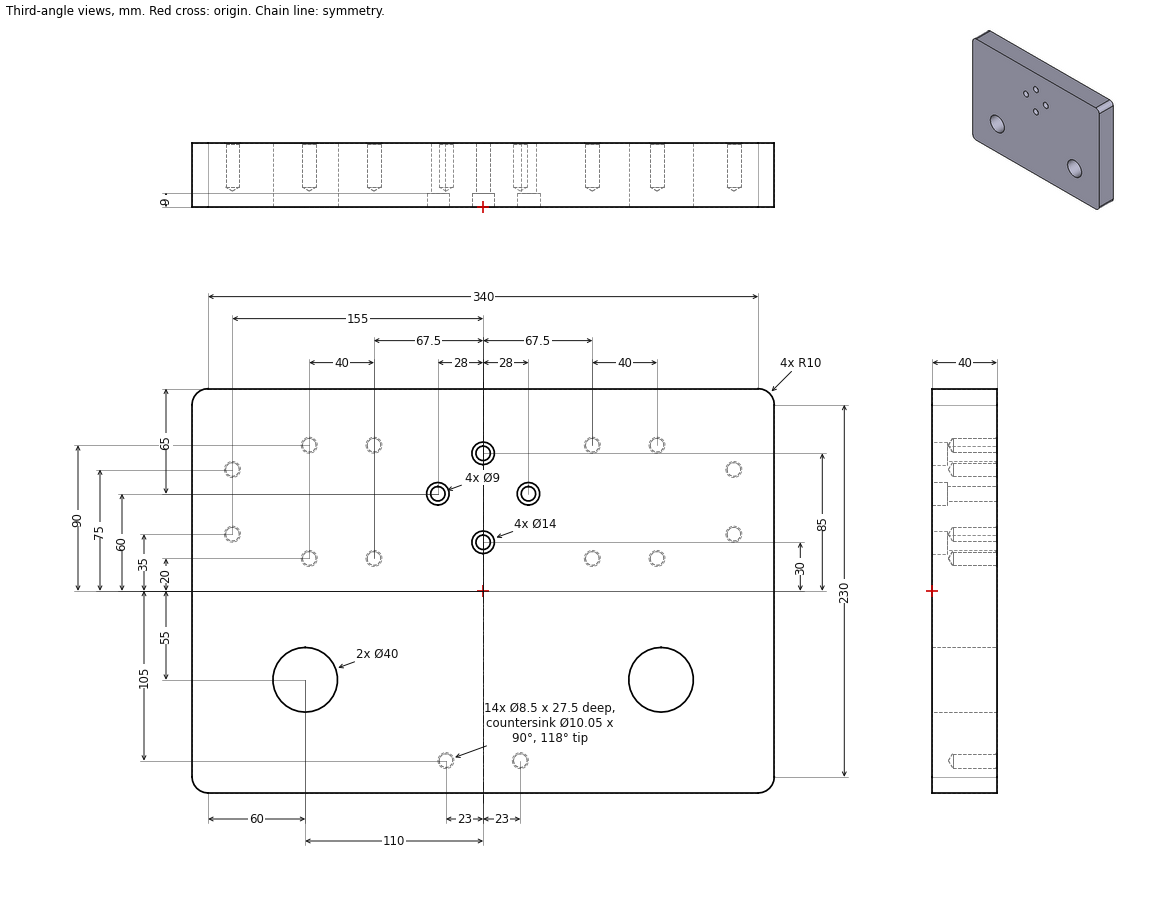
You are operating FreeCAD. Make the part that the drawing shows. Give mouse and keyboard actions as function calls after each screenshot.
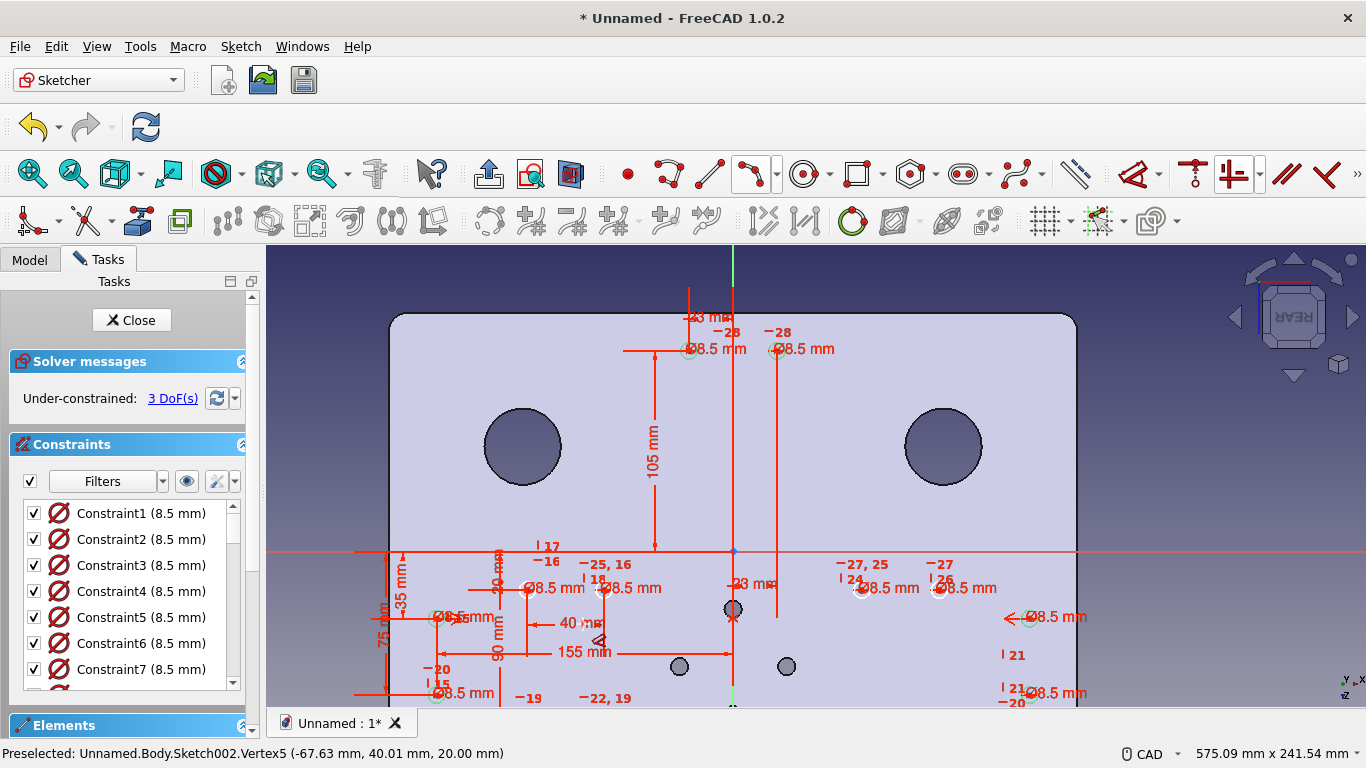
scroll(777, 351, down, 2)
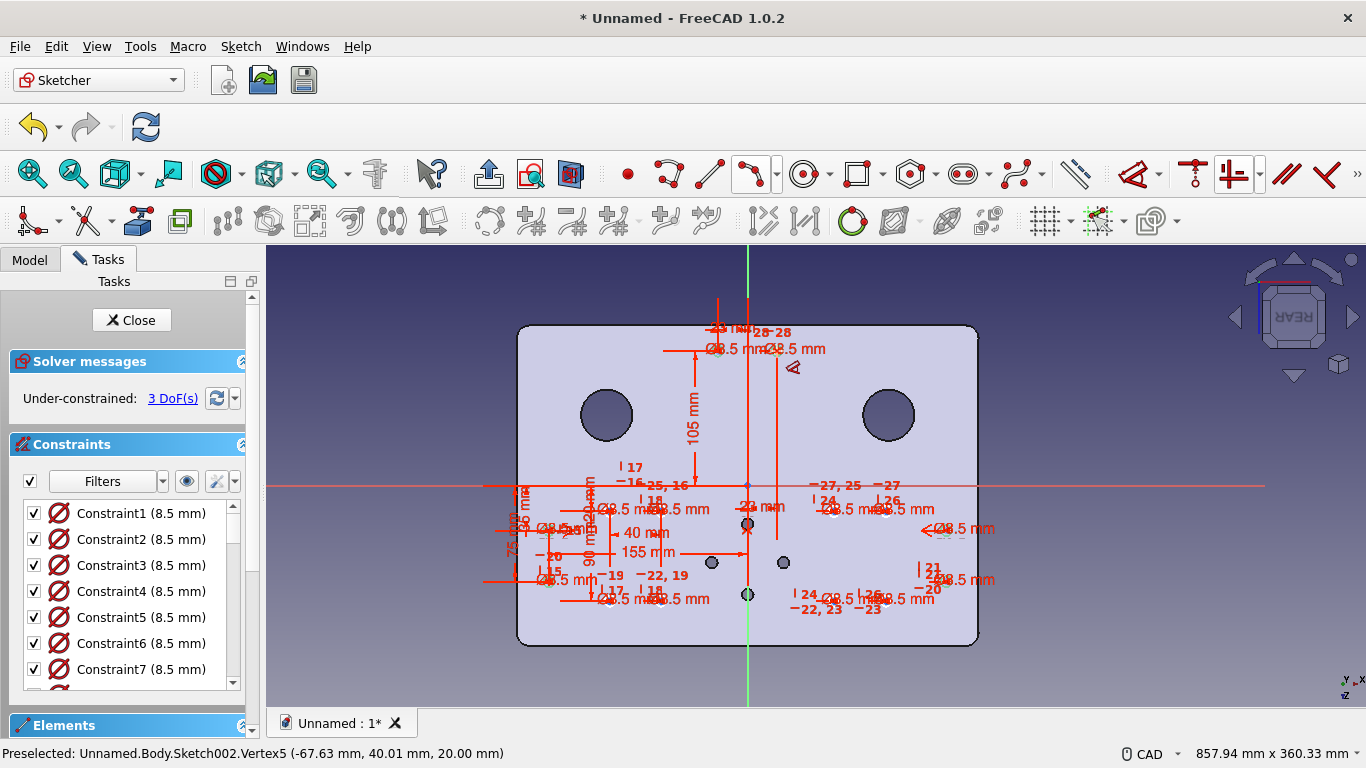
click(834, 601)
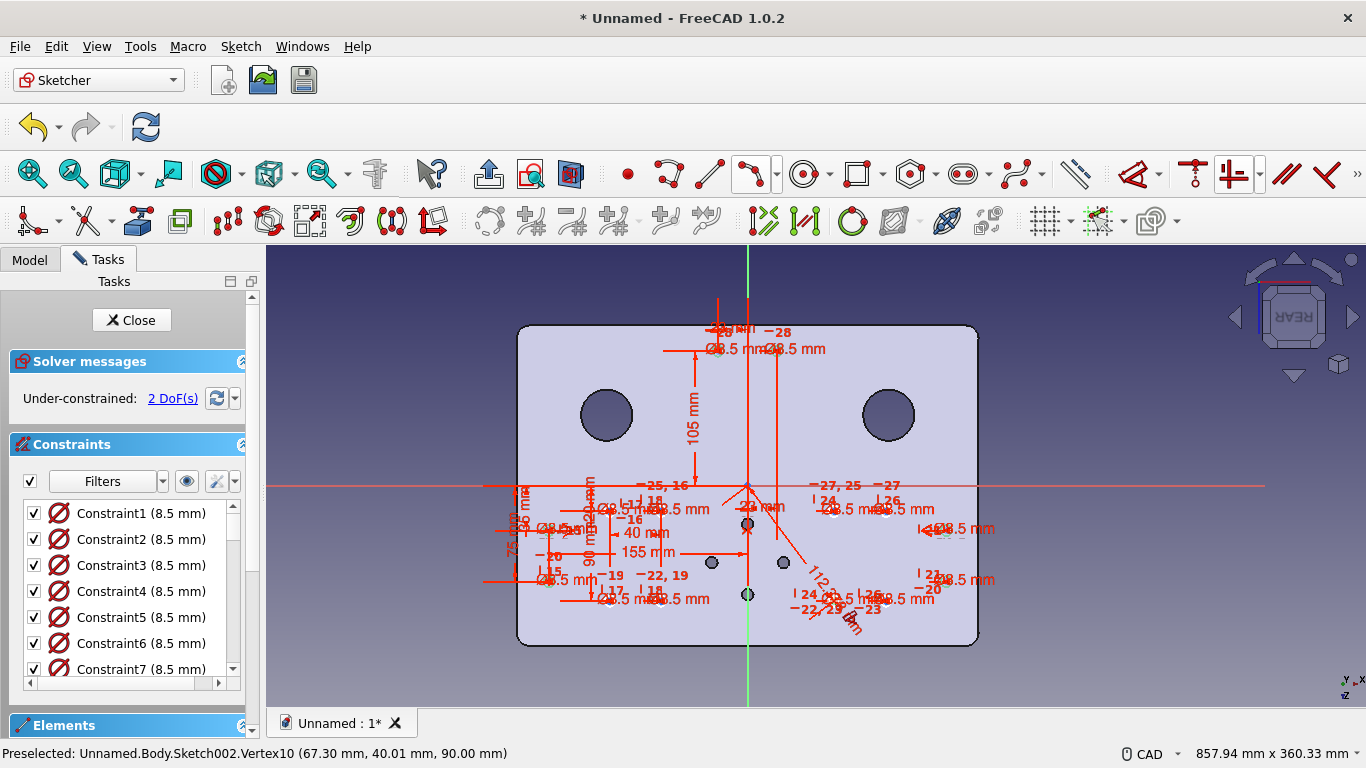
click(886, 601)
click(860, 635)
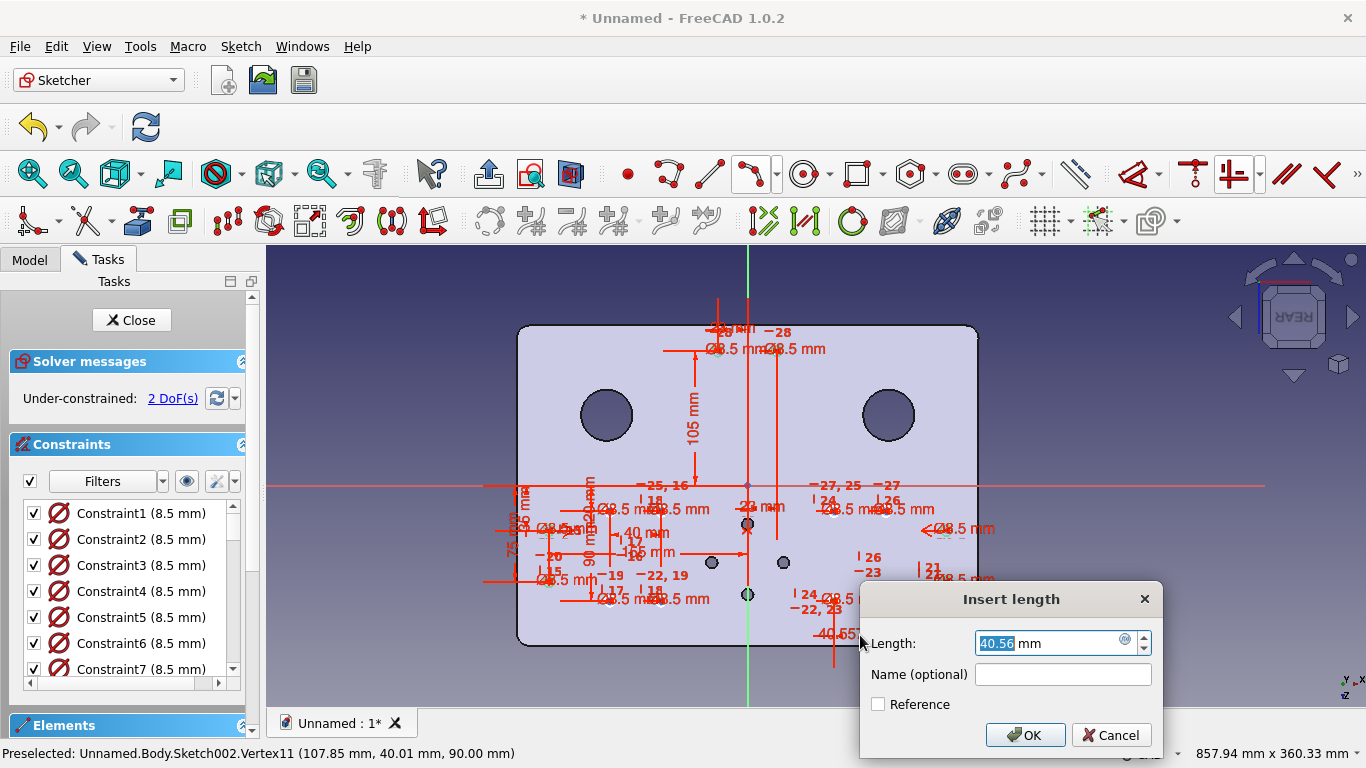
text(40)
key(Return)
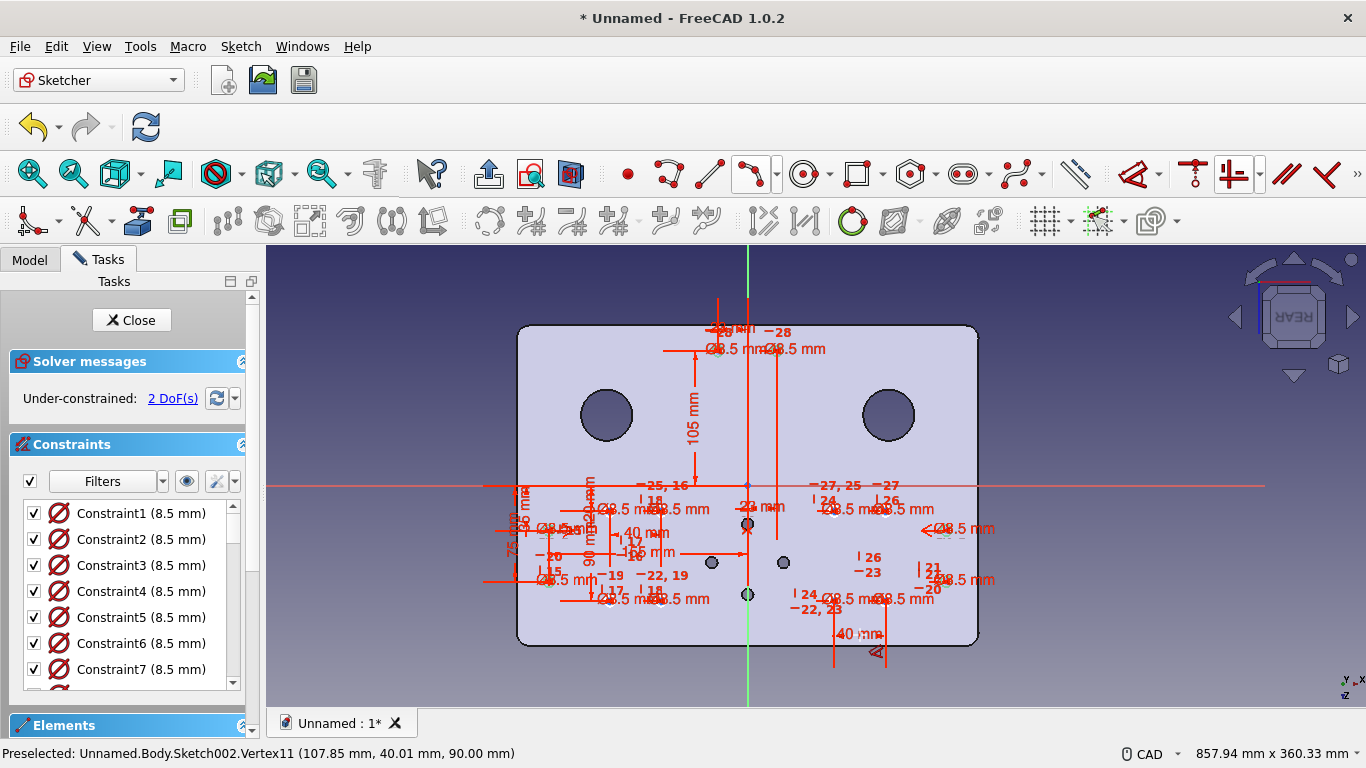
click(661, 511)
click(724, 545)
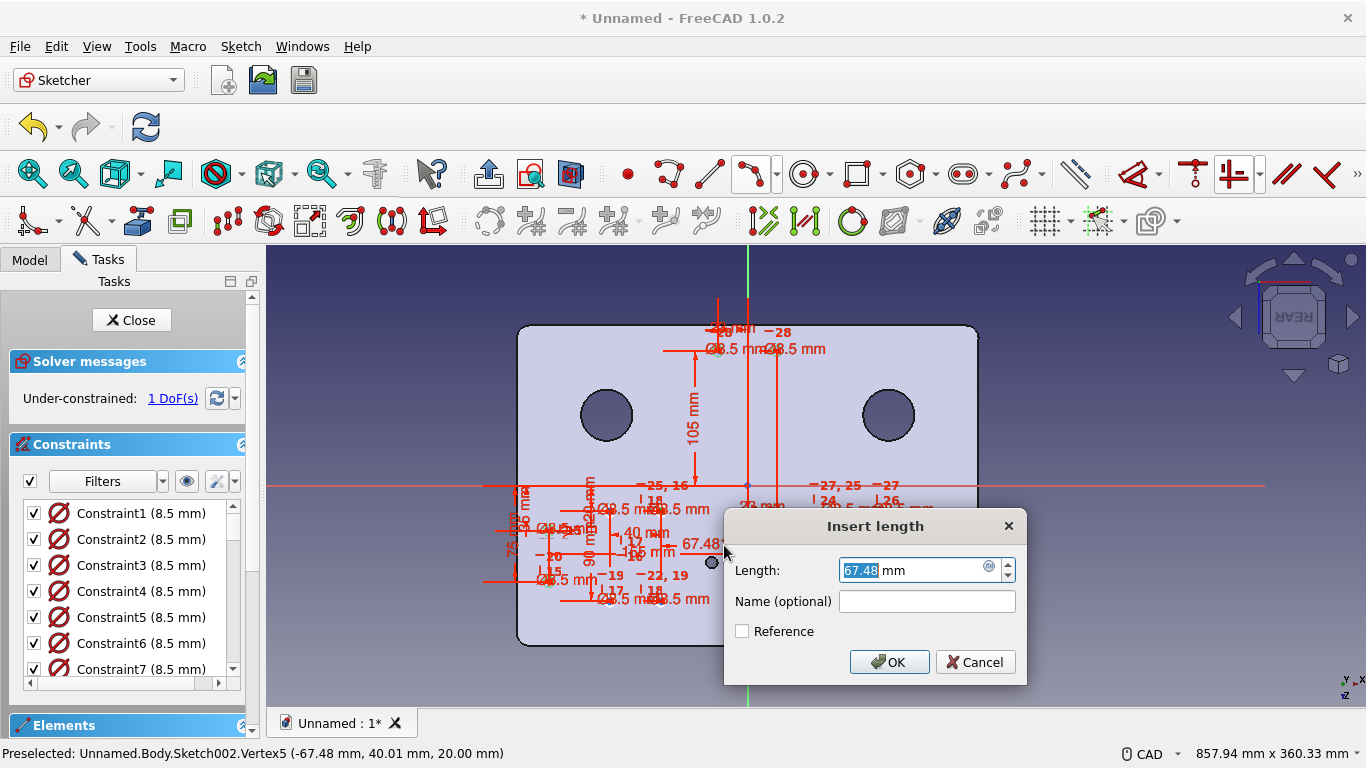
text(67.5)
key(Return)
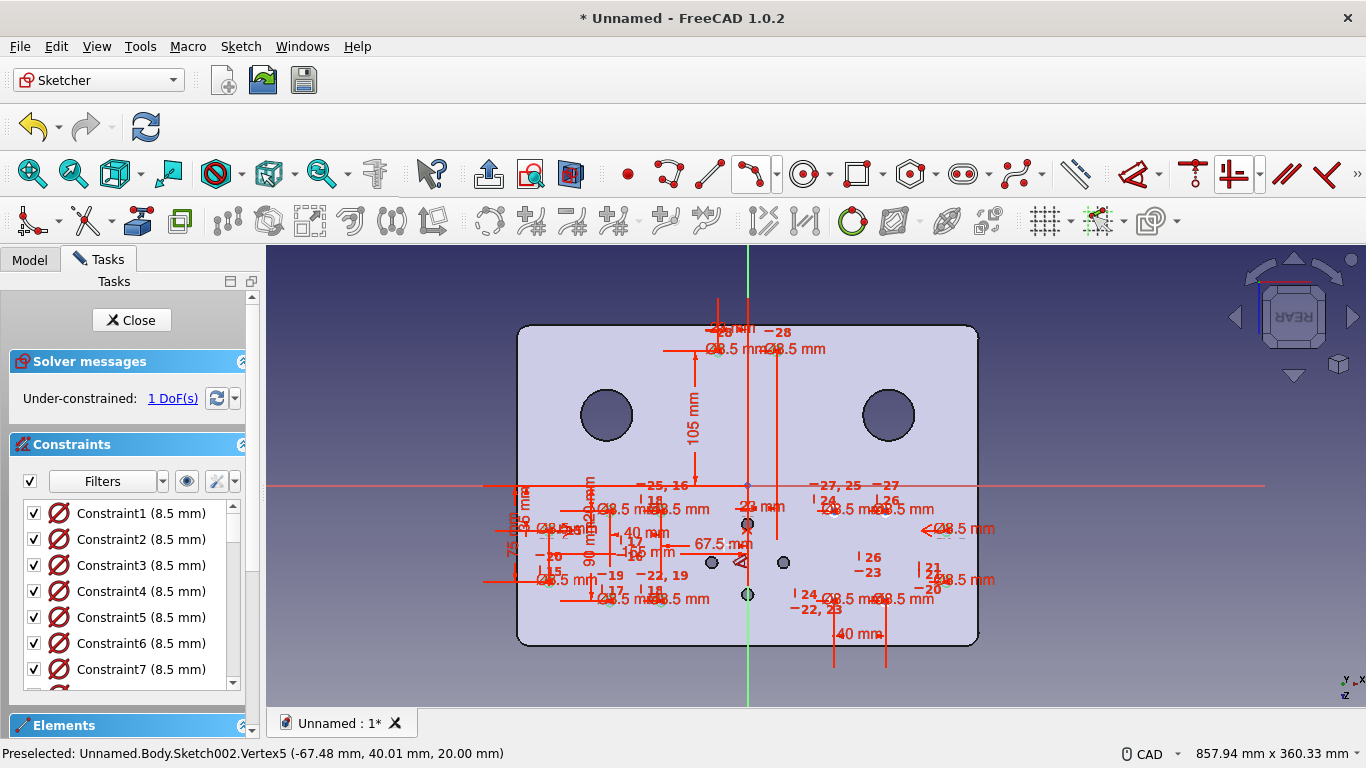
click(834, 601)
click(771, 635)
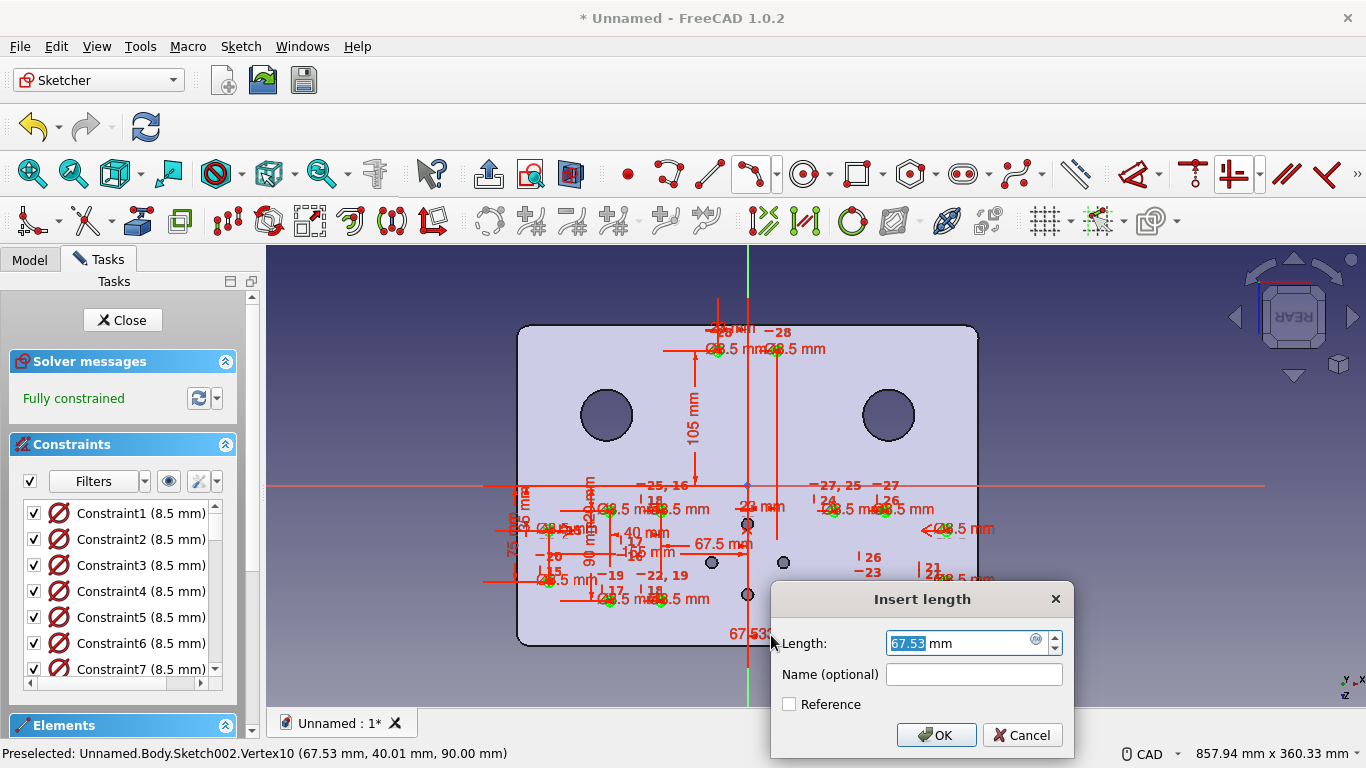
text(67.5)
key(Return)
key(Escape)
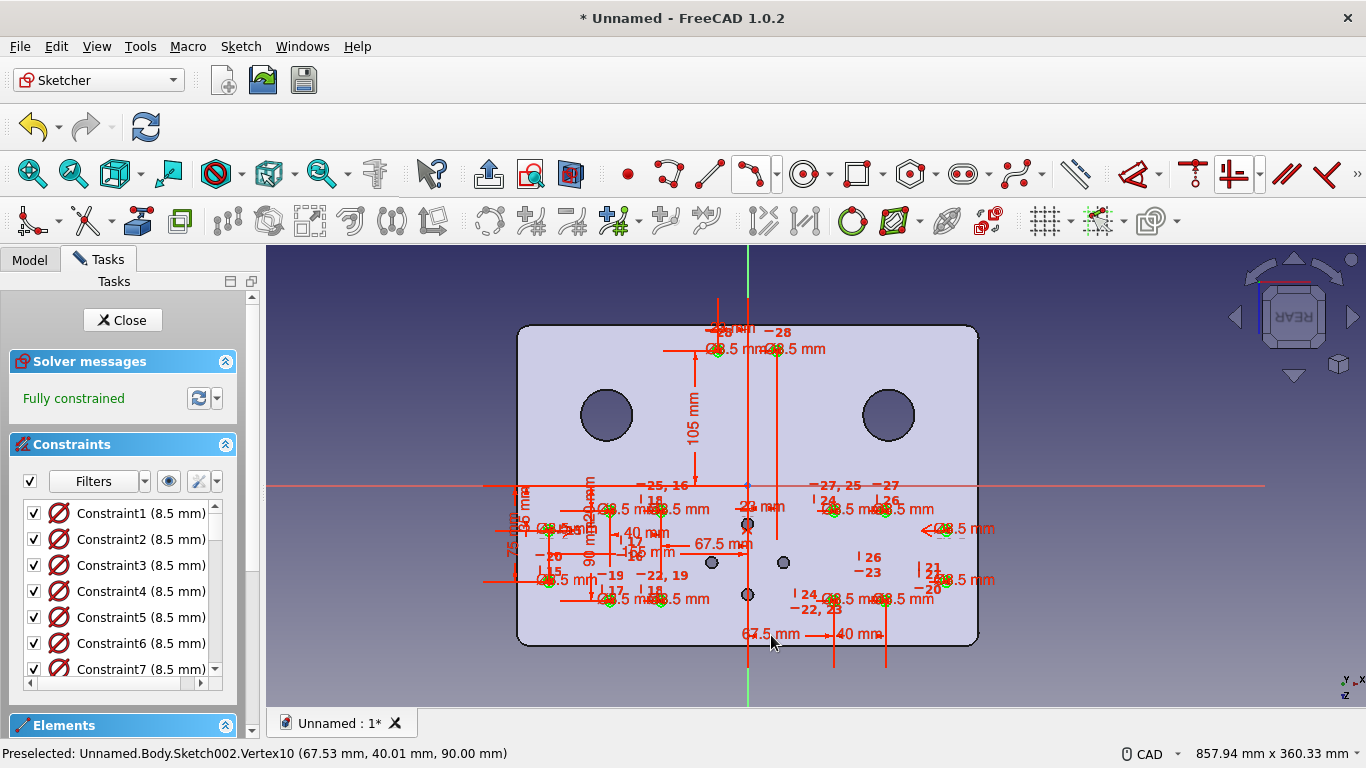
click(123, 320)